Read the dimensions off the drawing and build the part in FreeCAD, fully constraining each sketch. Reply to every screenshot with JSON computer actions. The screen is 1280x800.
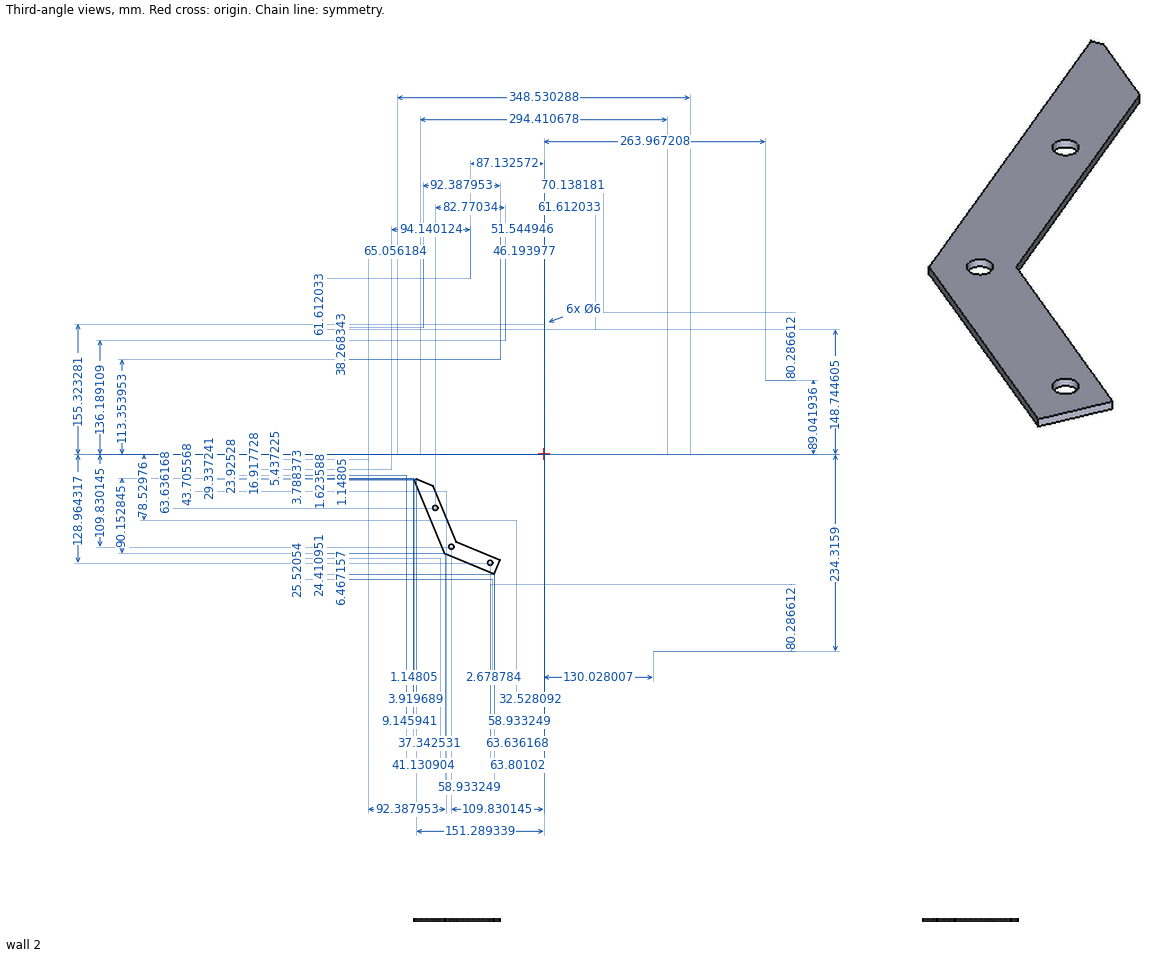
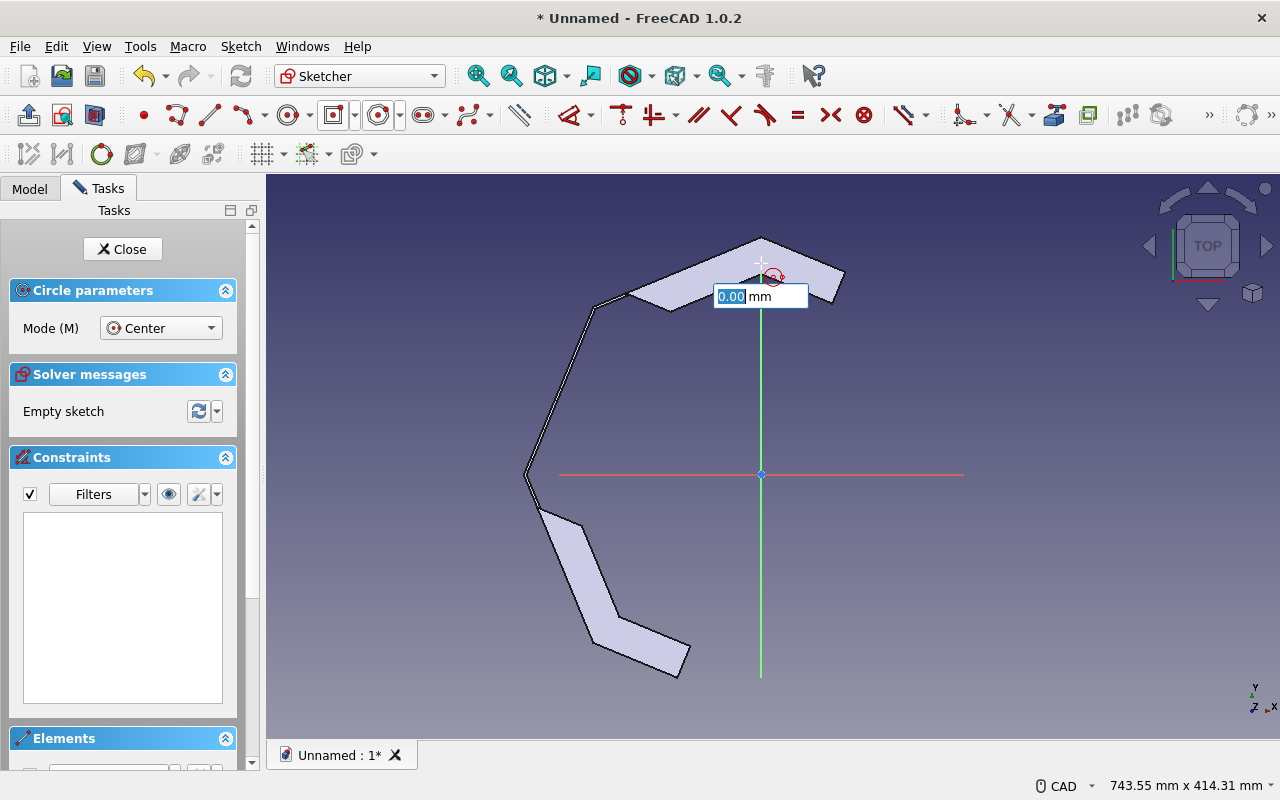
{"action": "scroll", "coordinate": [765, 262], "scroll_direction": "up", "scroll_amount": 8}
{"action": "mouse_move", "coordinate": [764, 260]}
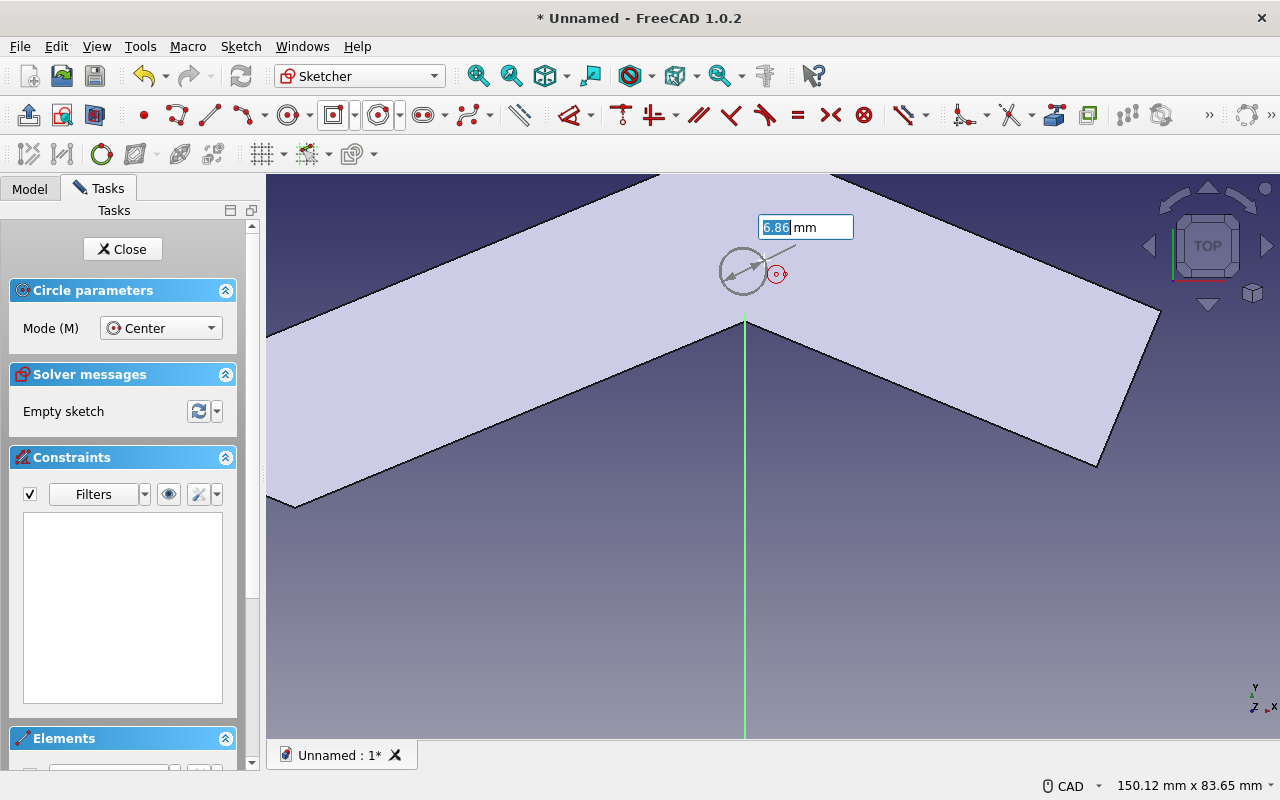
{"action": "type", "text": "6"}
{"action": "key", "text": "Return"}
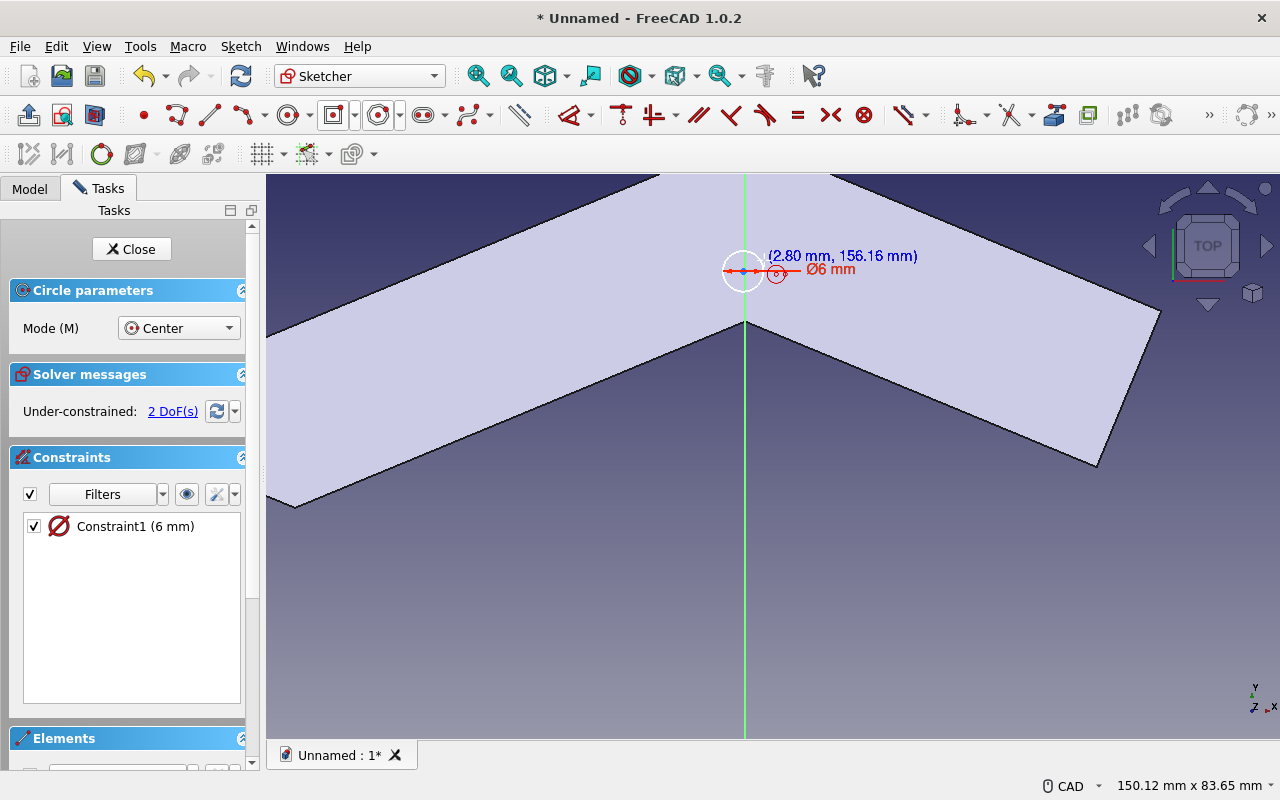
{"action": "scroll", "coordinate": [765, 262], "scroll_direction": "down", "scroll_amount": 8}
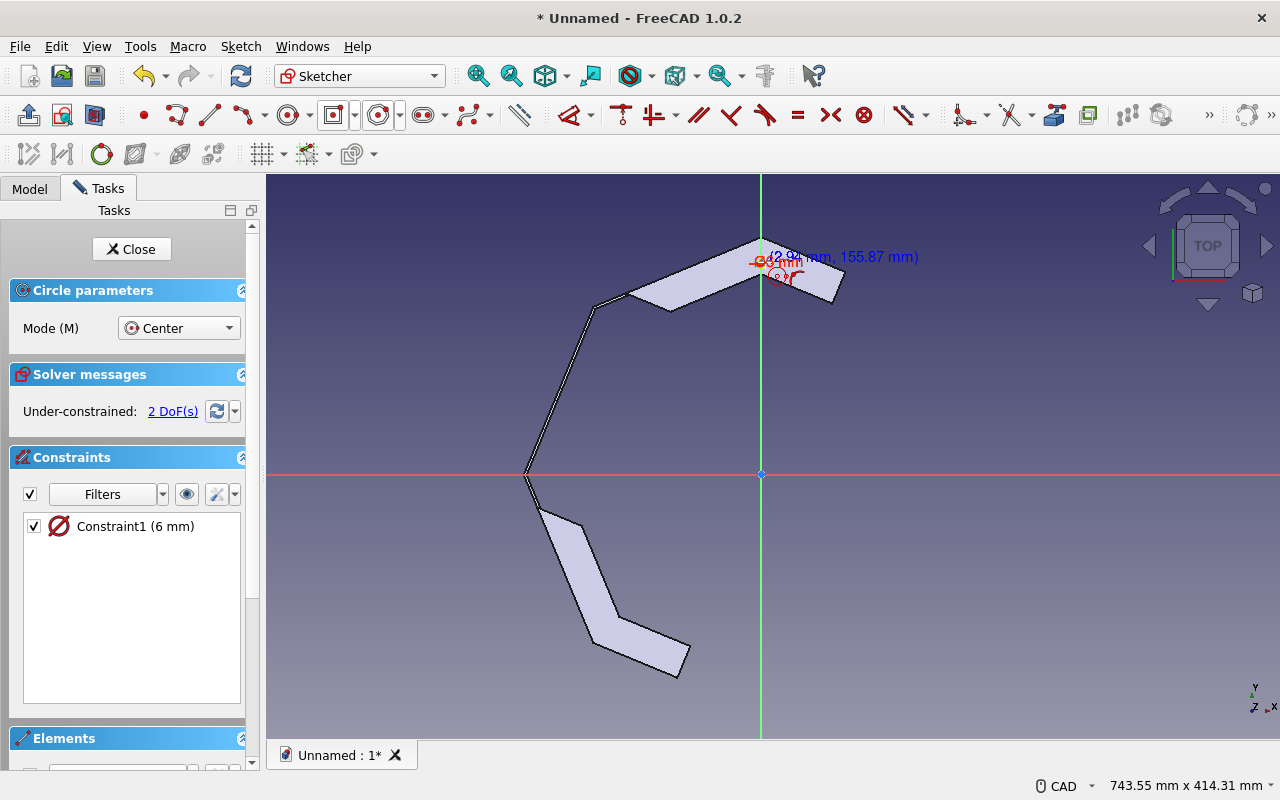
{"action": "left_click", "coordinate": [698, 289]}
{"action": "mouse_move", "coordinate": [701, 286]}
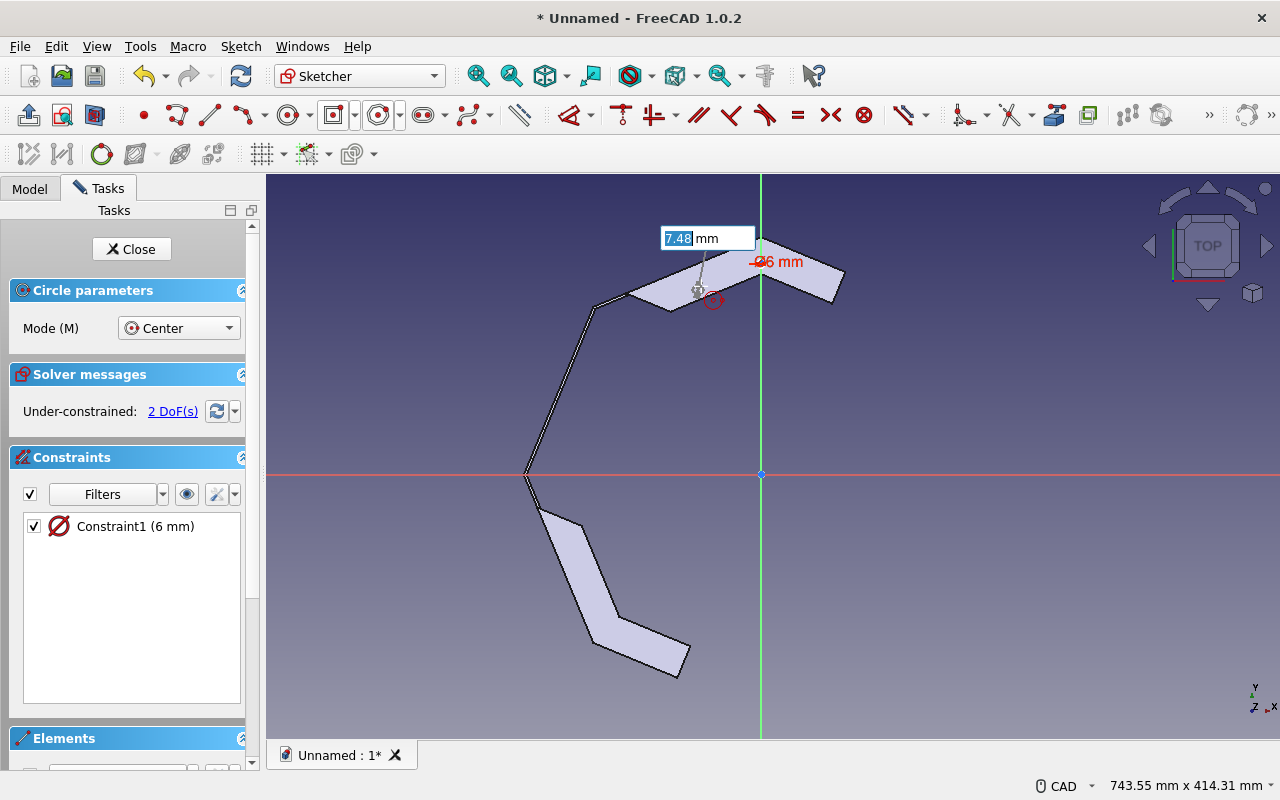
{"action": "type", "text": "6"}
{"action": "key", "text": "Return"}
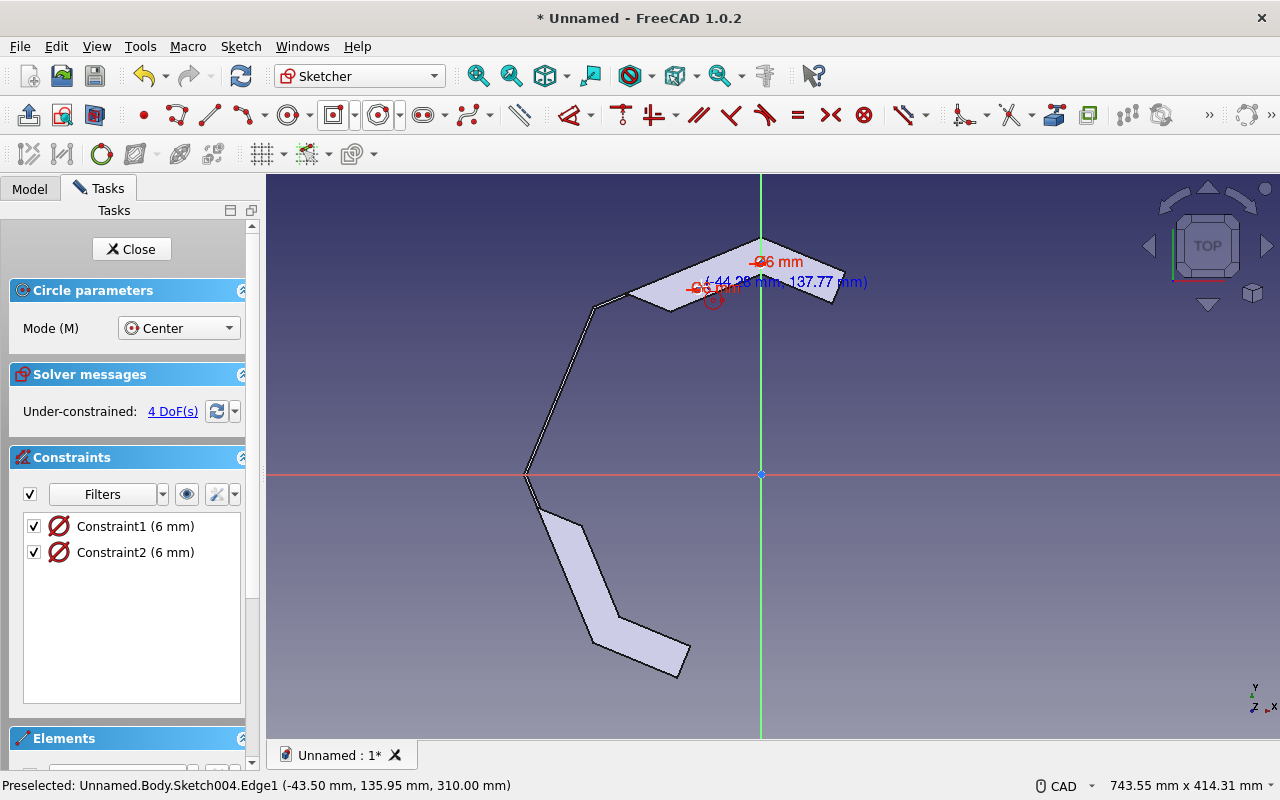
{"action": "scroll", "coordinate": [824, 289], "scroll_direction": "up", "scroll_amount": 9}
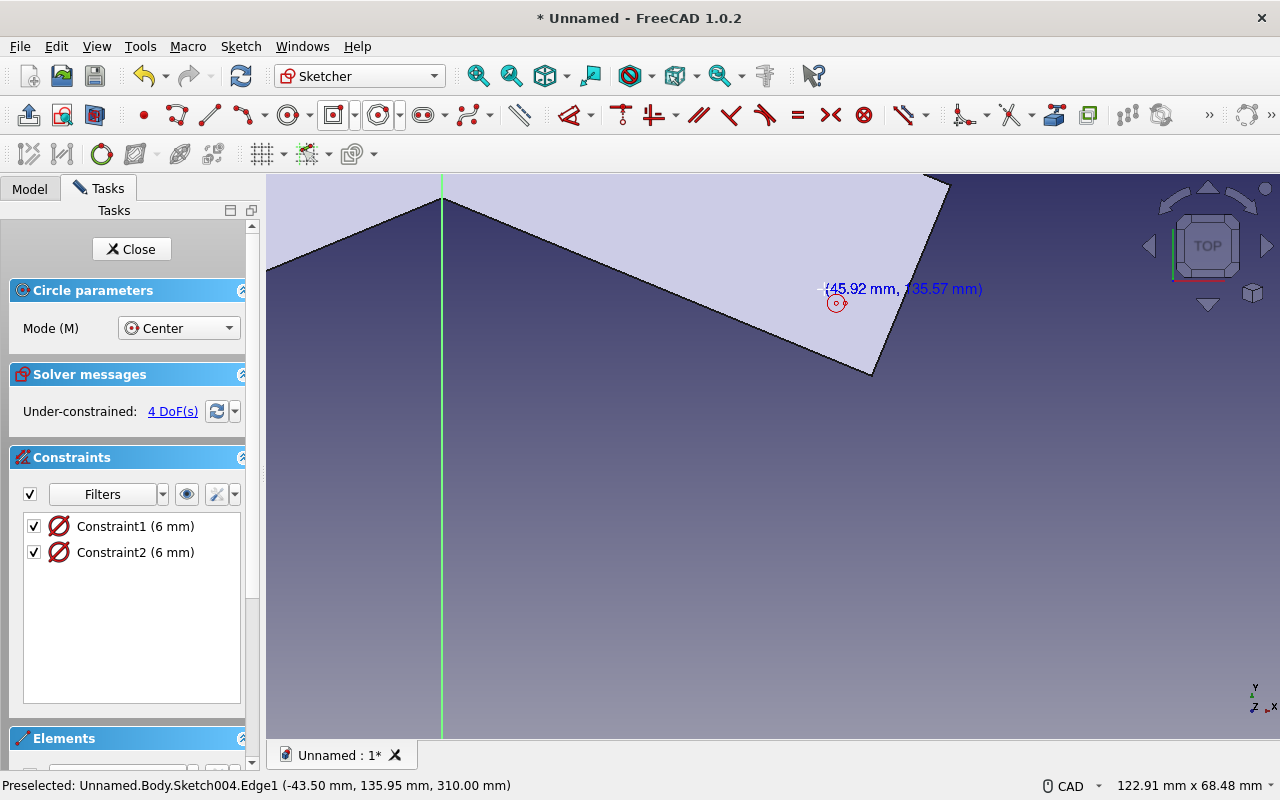
{"action": "scroll", "coordinate": [824, 289], "scroll_direction": "down", "scroll_amount": 9}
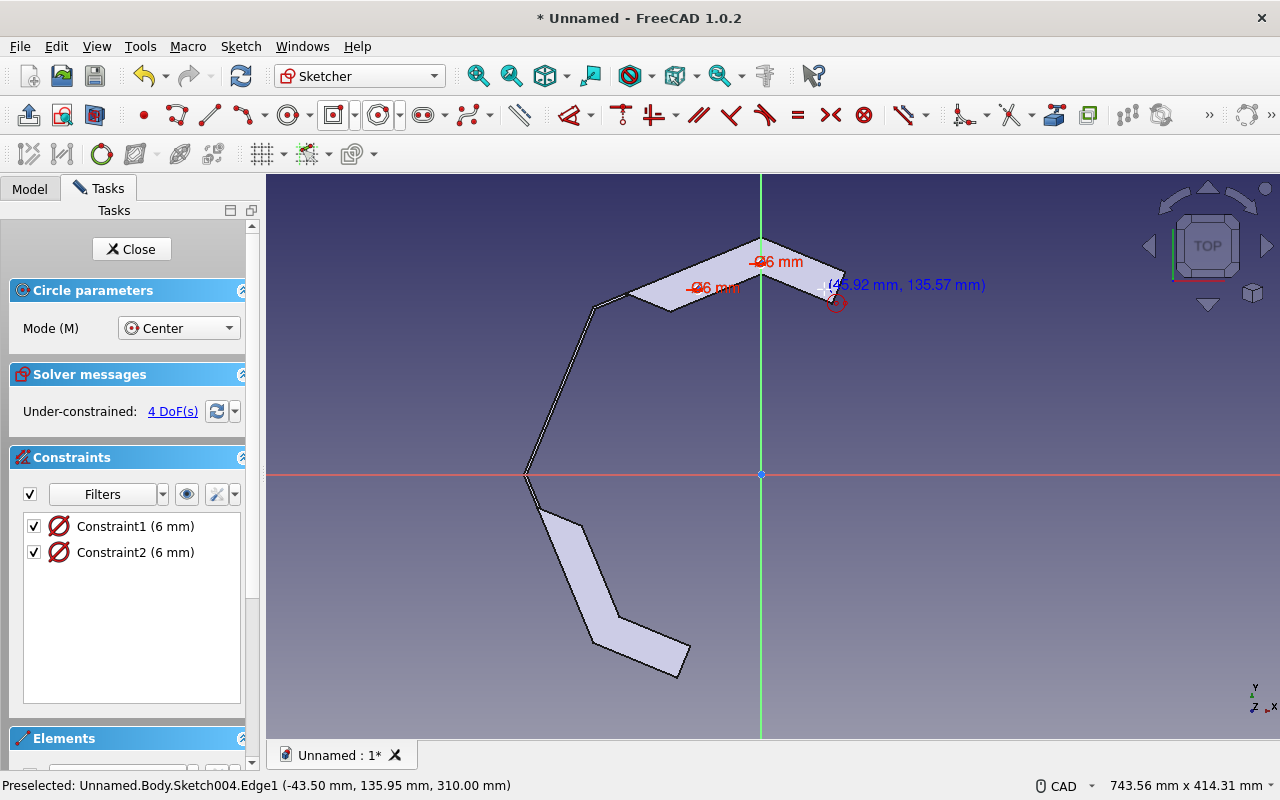
{"action": "left_click", "coordinate": [824, 289]}
{"action": "mouse_move", "coordinate": [827, 286]}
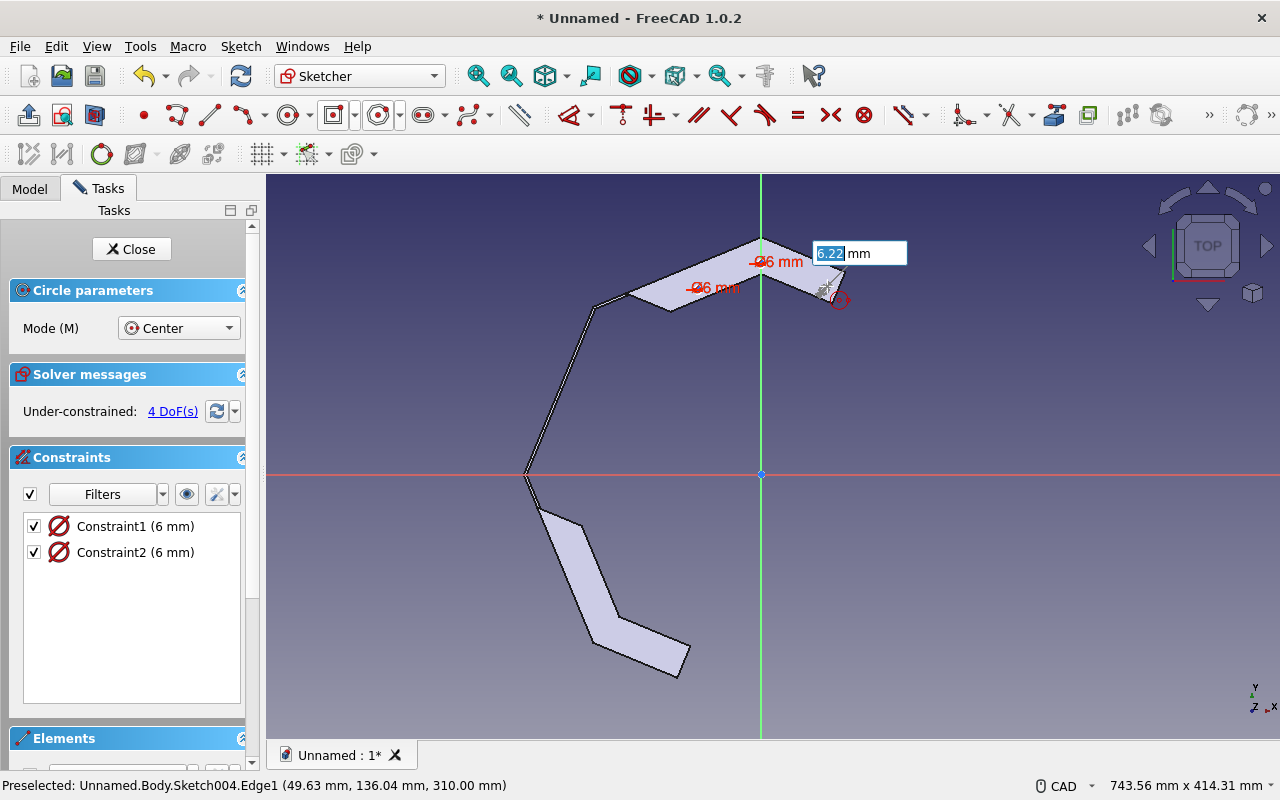
{"action": "type", "text": "6"}
{"action": "key", "text": "Return"}